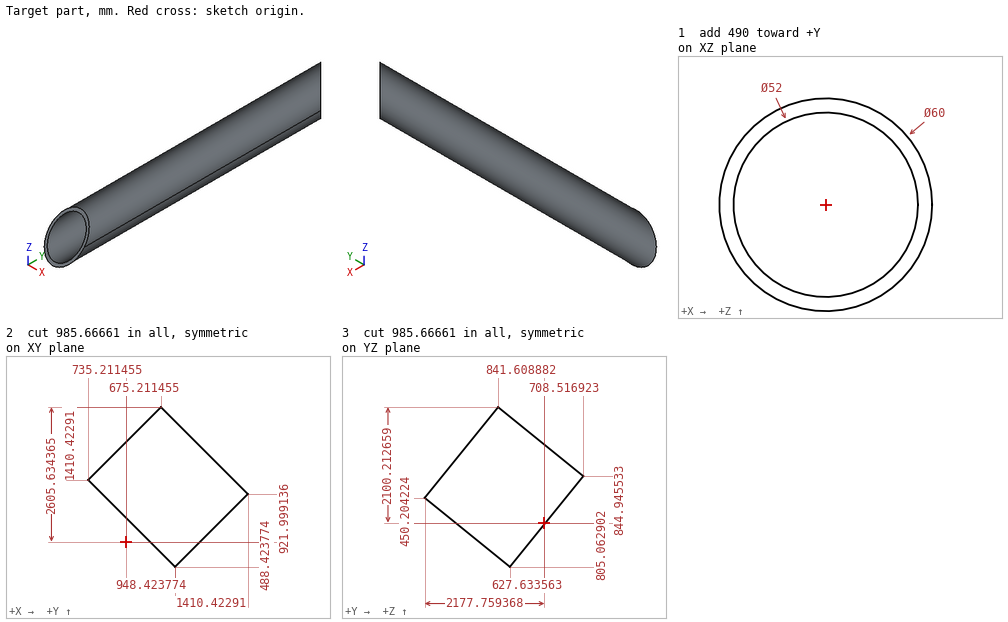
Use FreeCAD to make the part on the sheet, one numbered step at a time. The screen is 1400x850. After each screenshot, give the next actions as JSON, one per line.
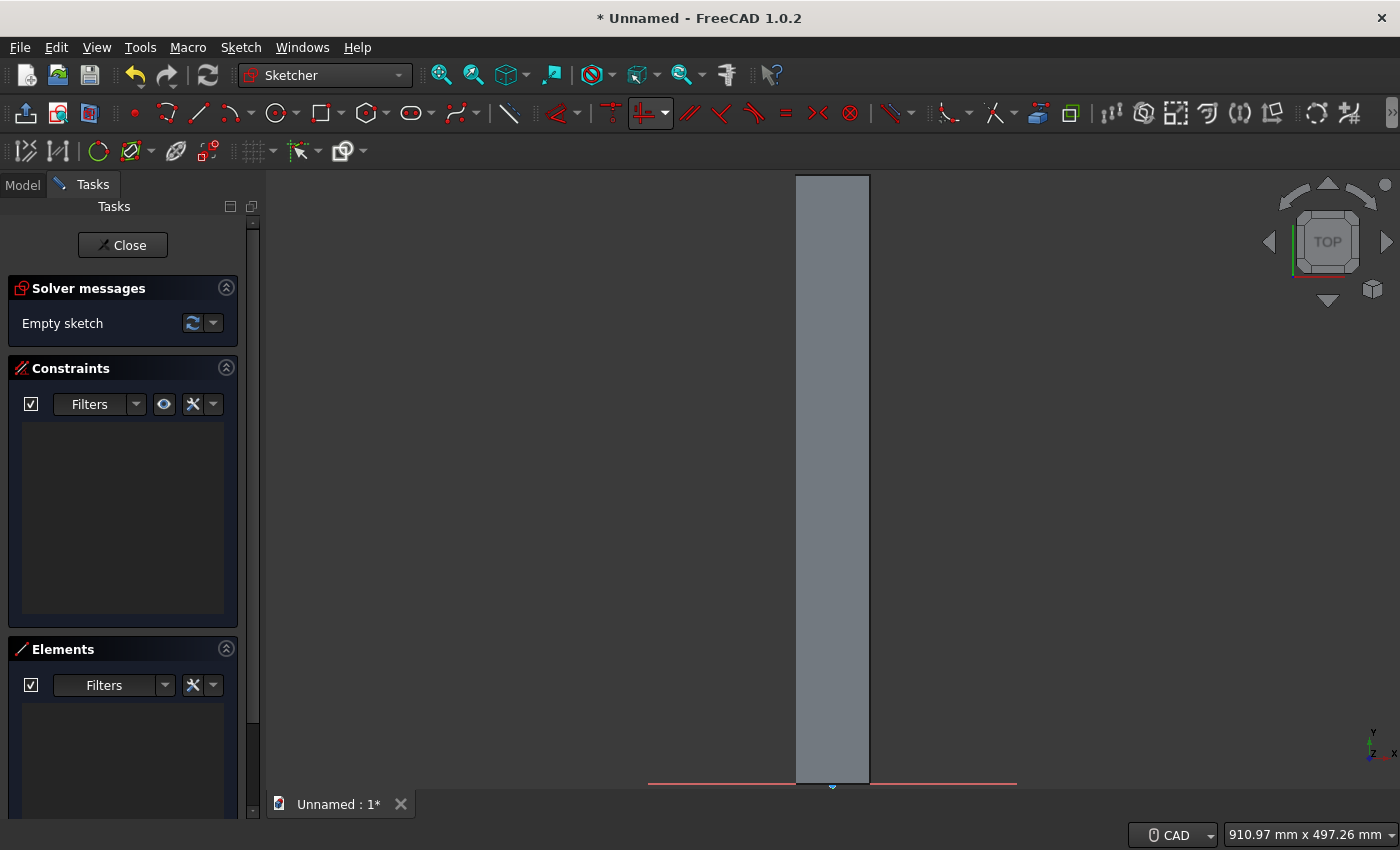
{"action": "left_click", "coordinate": [90, 114]}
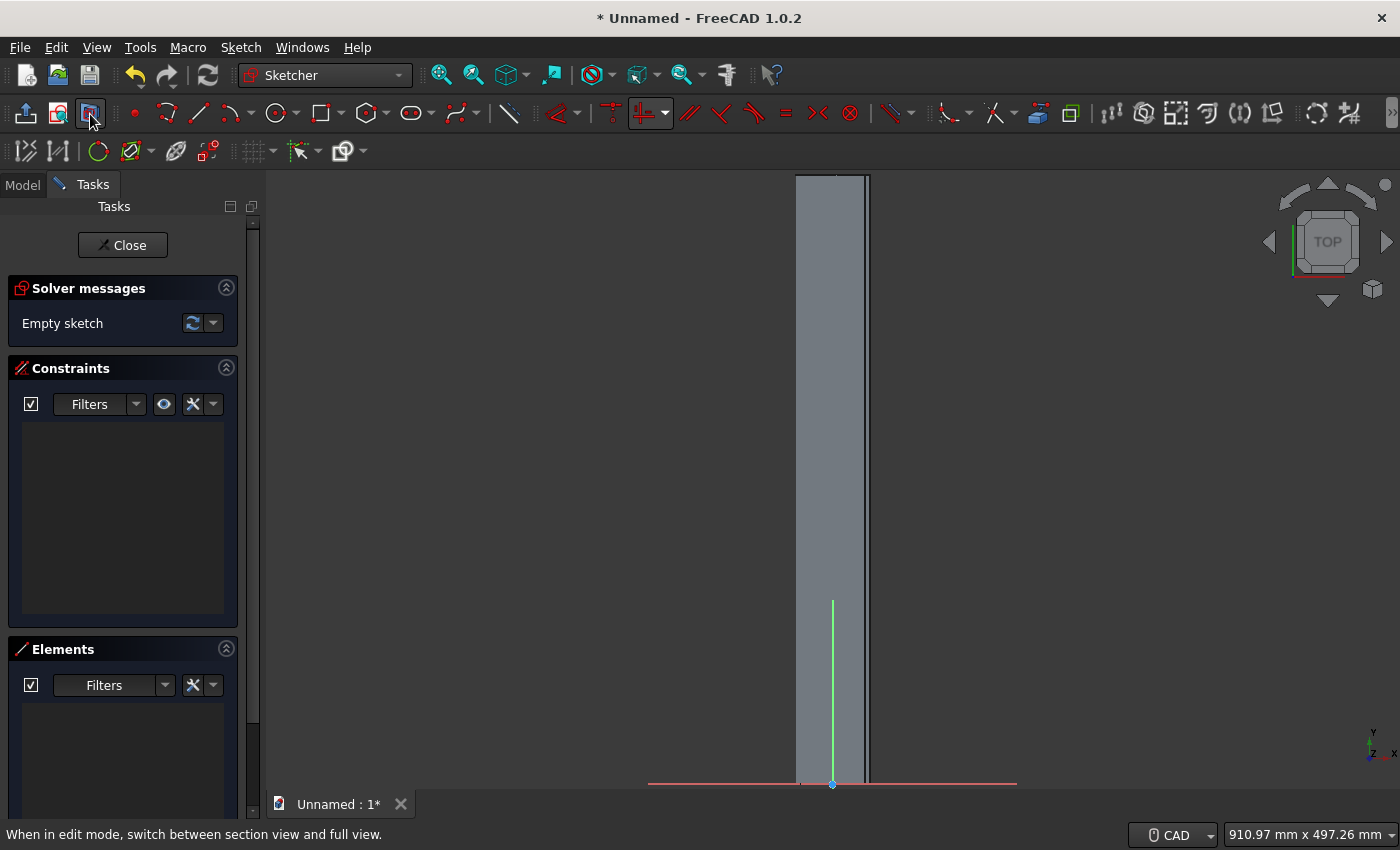
{"action": "scroll", "coordinate": [630, 606], "scroll_direction": "down", "scroll_amount": 11}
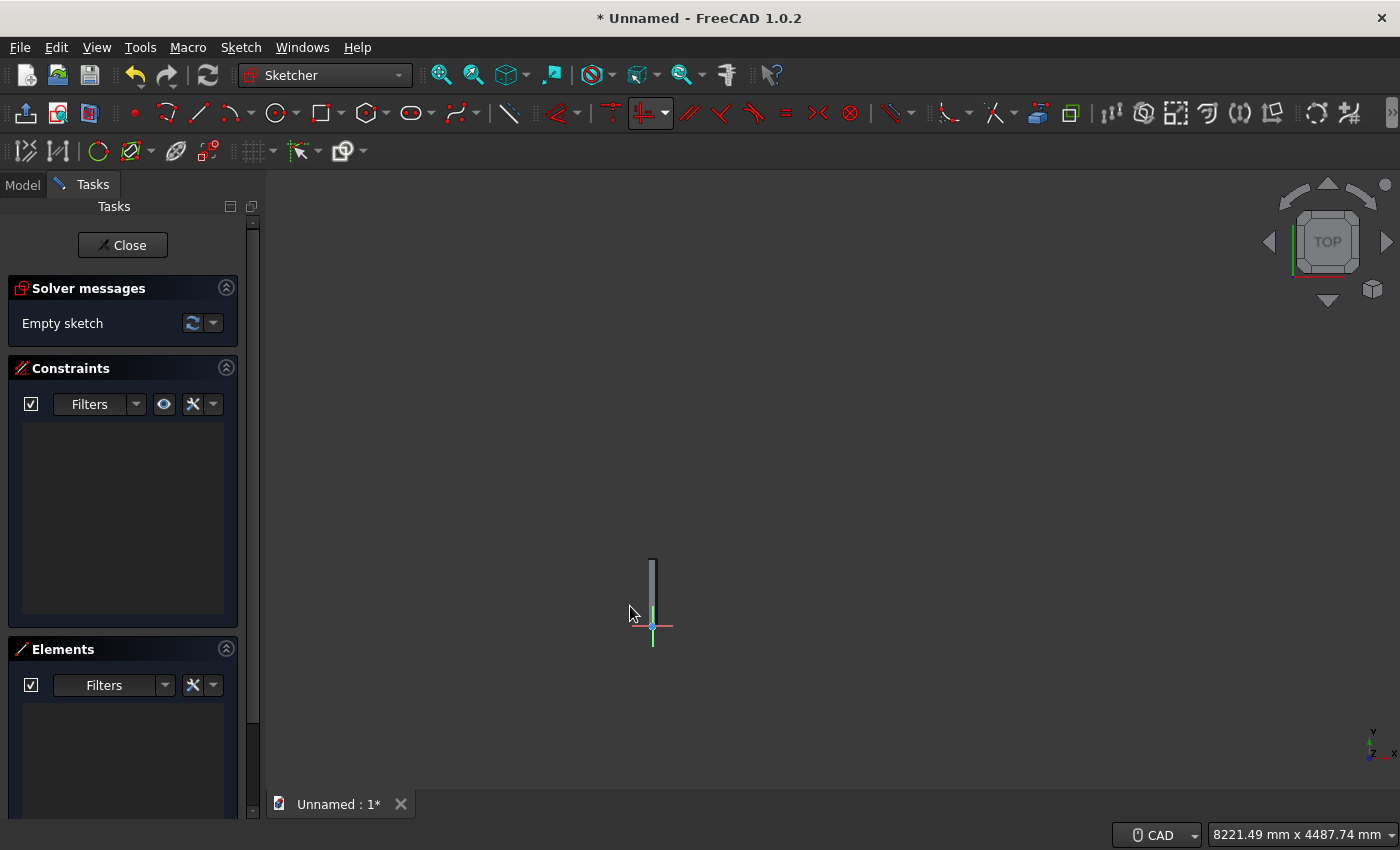
{"action": "key", "text": "g m"}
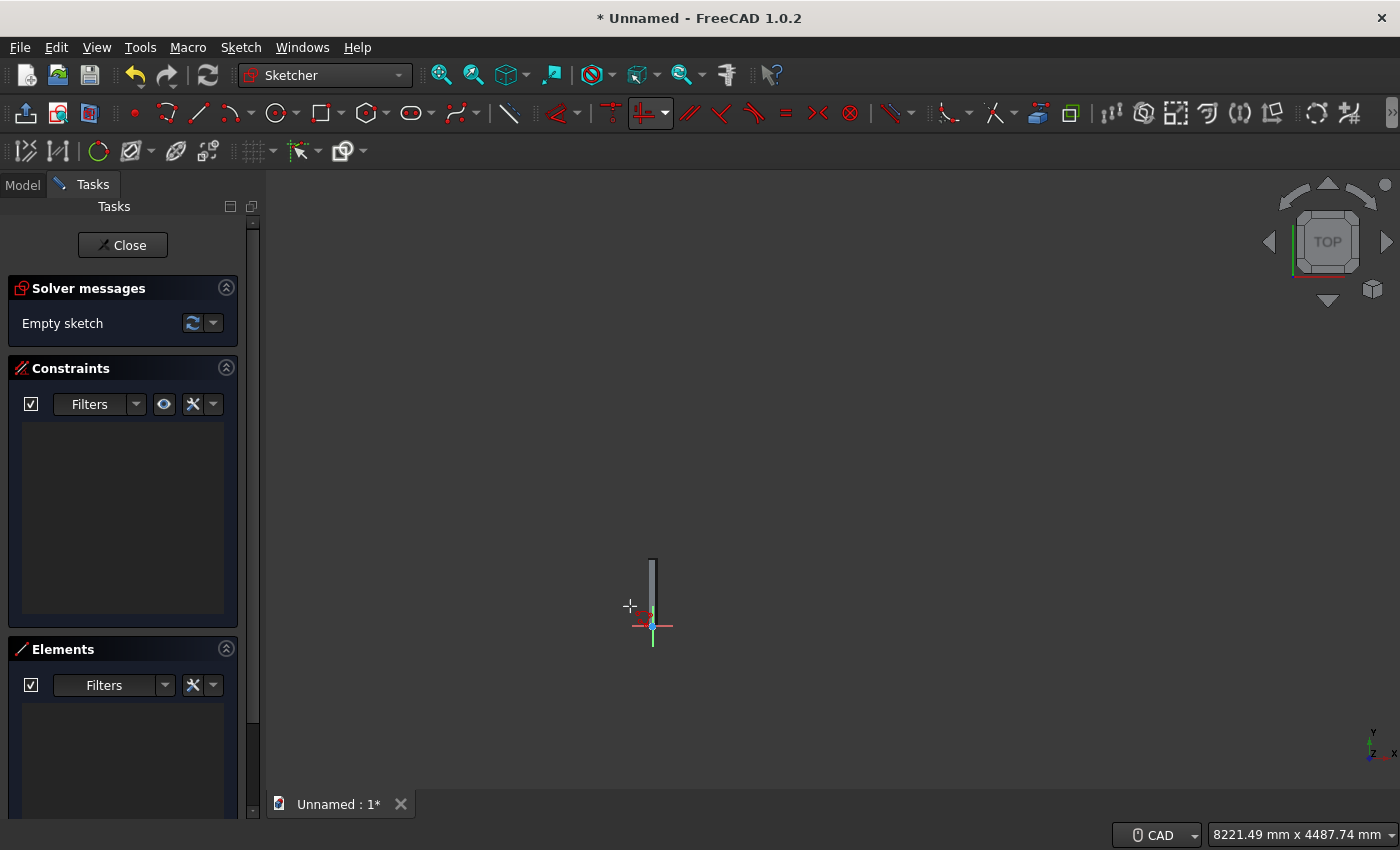
{"action": "left_click", "coordinate": [784, 694]}
{"action": "left_click", "coordinate": [978, 499]}
{"action": "left_click", "coordinate": [746, 267]}
{"action": "left_click", "coordinate": [551, 462]}
{"action": "left_click", "coordinate": [784, 695]}
{"action": "key", "text": "Escape"}
{"action": "key", "text": "Escape"}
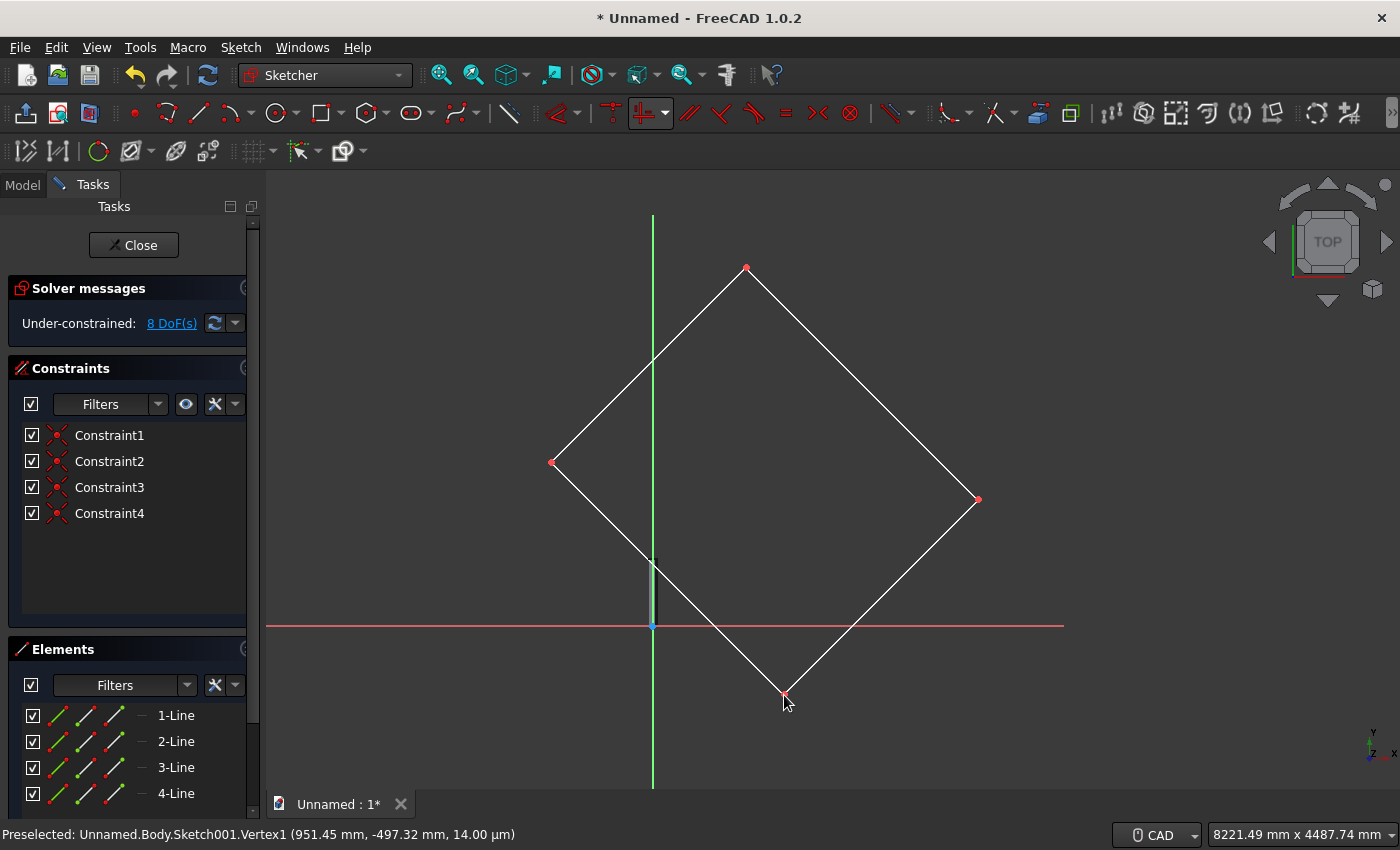
{"action": "left_click", "coordinate": [556, 114]}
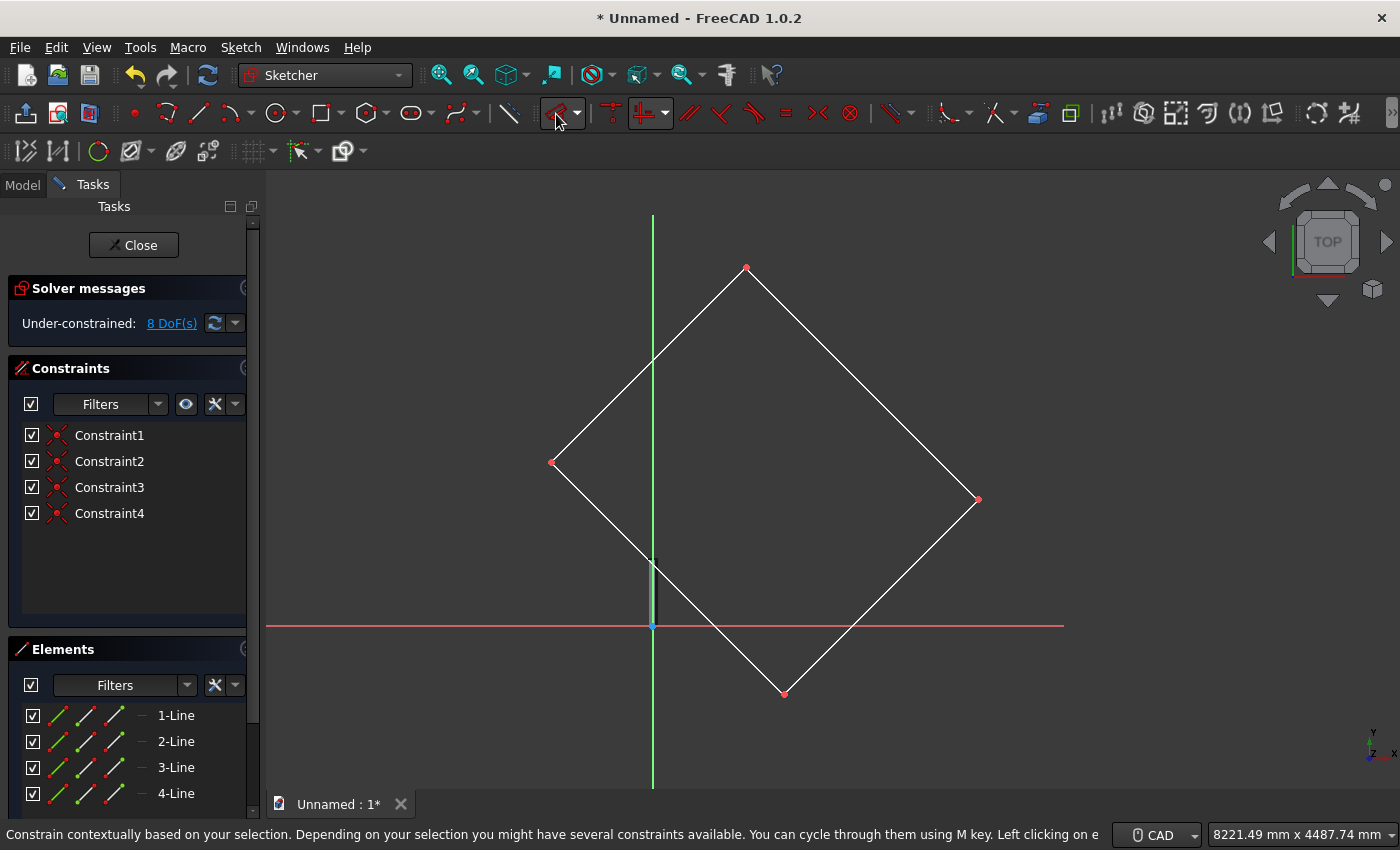
{"action": "left_click", "coordinate": [784, 695]}
{"action": "left_click", "coordinate": [718, 729]}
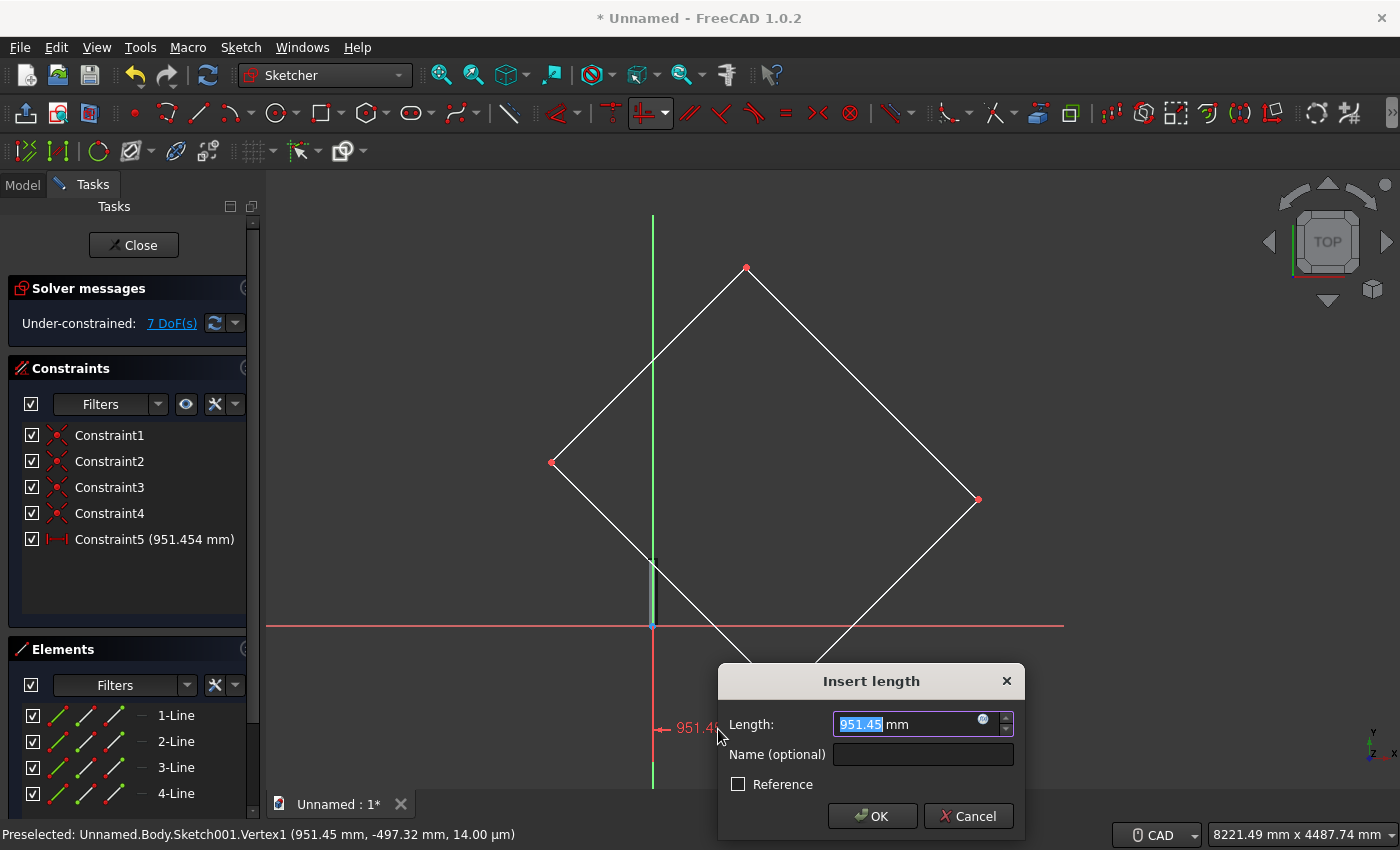
{"action": "type", "text": "948.423774"}
{"action": "key", "text": "Return"}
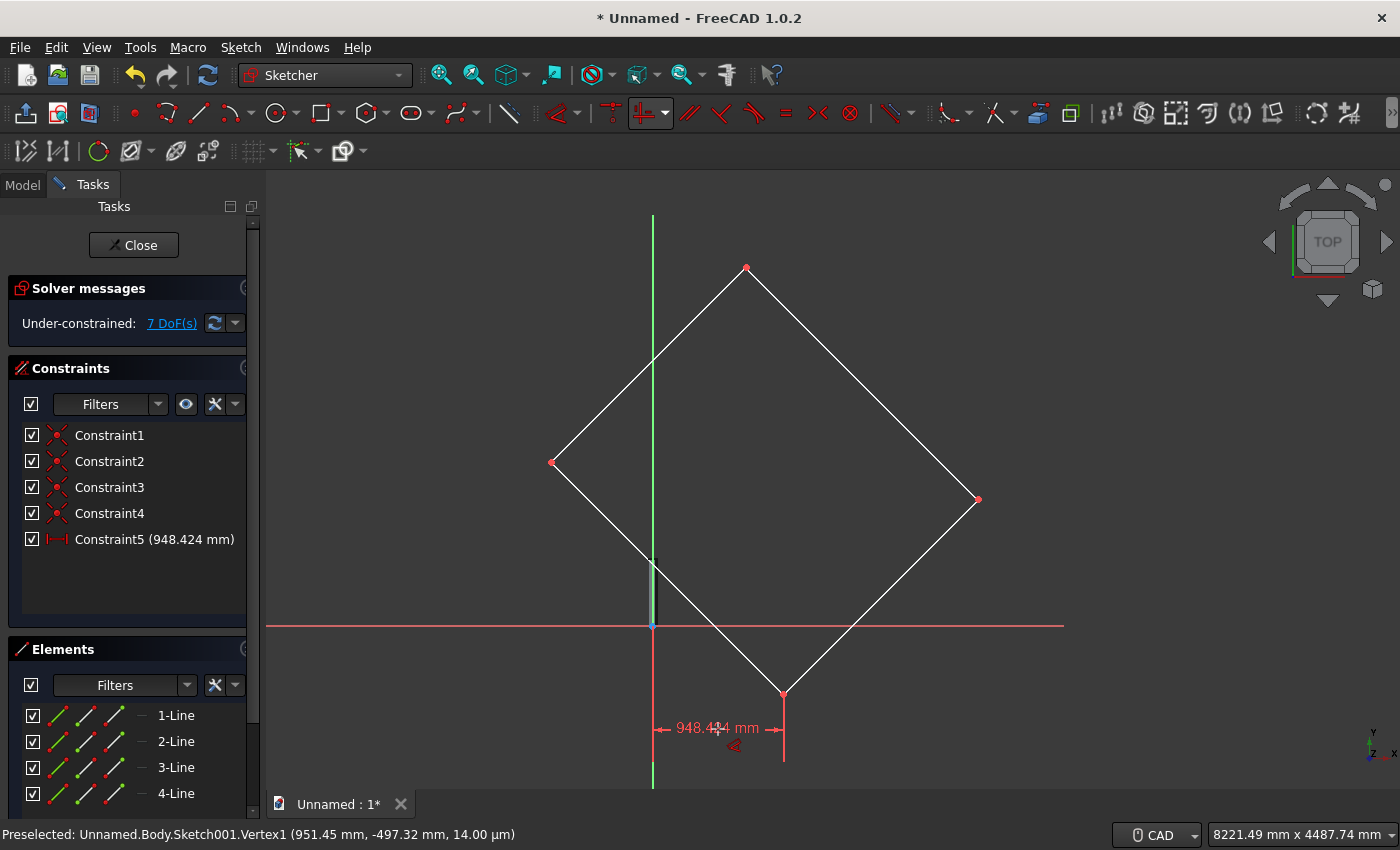
{"action": "left_click", "coordinate": [784, 695]}
{"action": "left_click", "coordinate": [619, 661]}